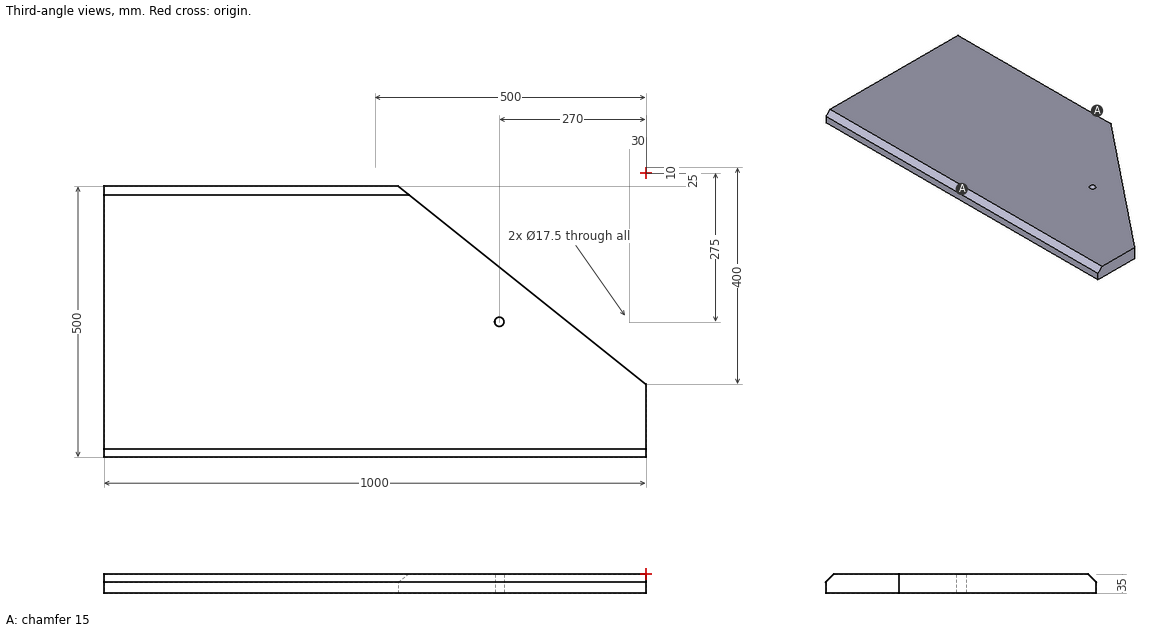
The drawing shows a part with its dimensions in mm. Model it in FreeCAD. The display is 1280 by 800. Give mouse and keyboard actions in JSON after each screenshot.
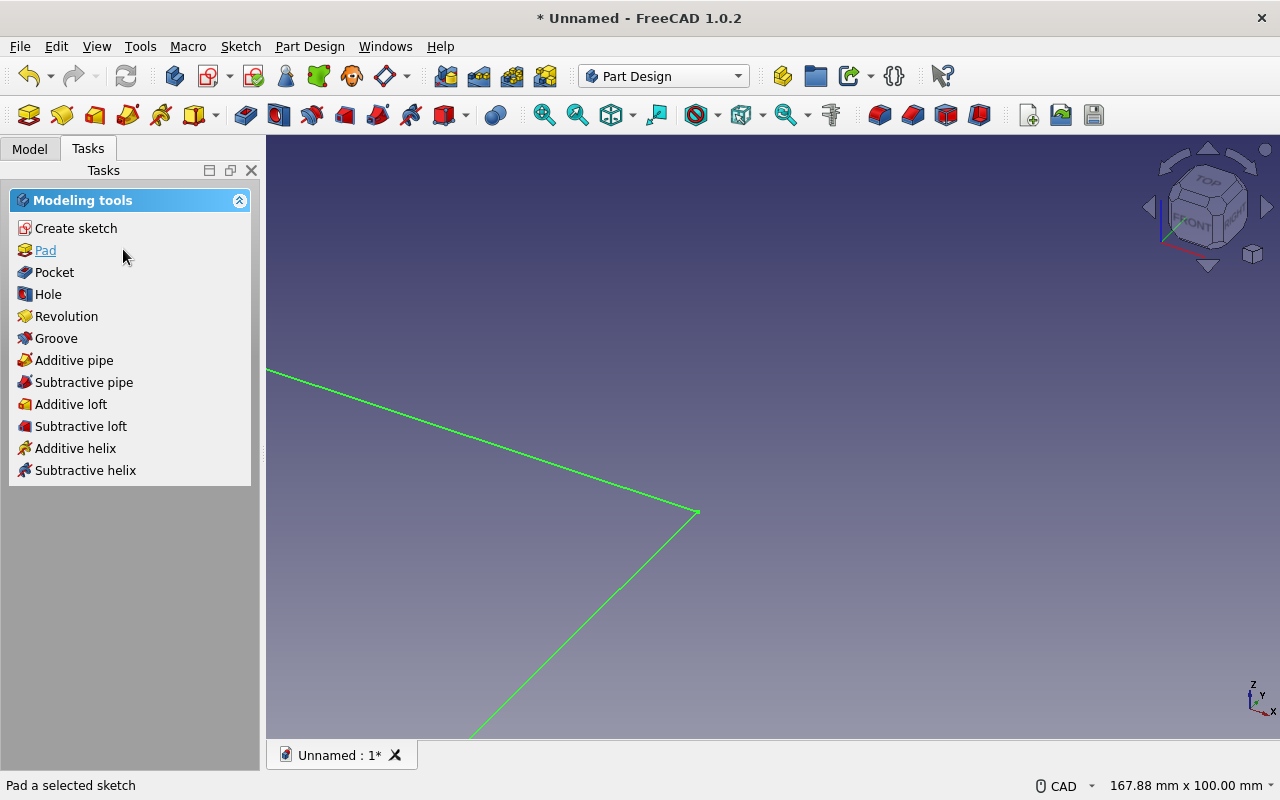
{"action": "left_click", "coordinate": [29, 116]}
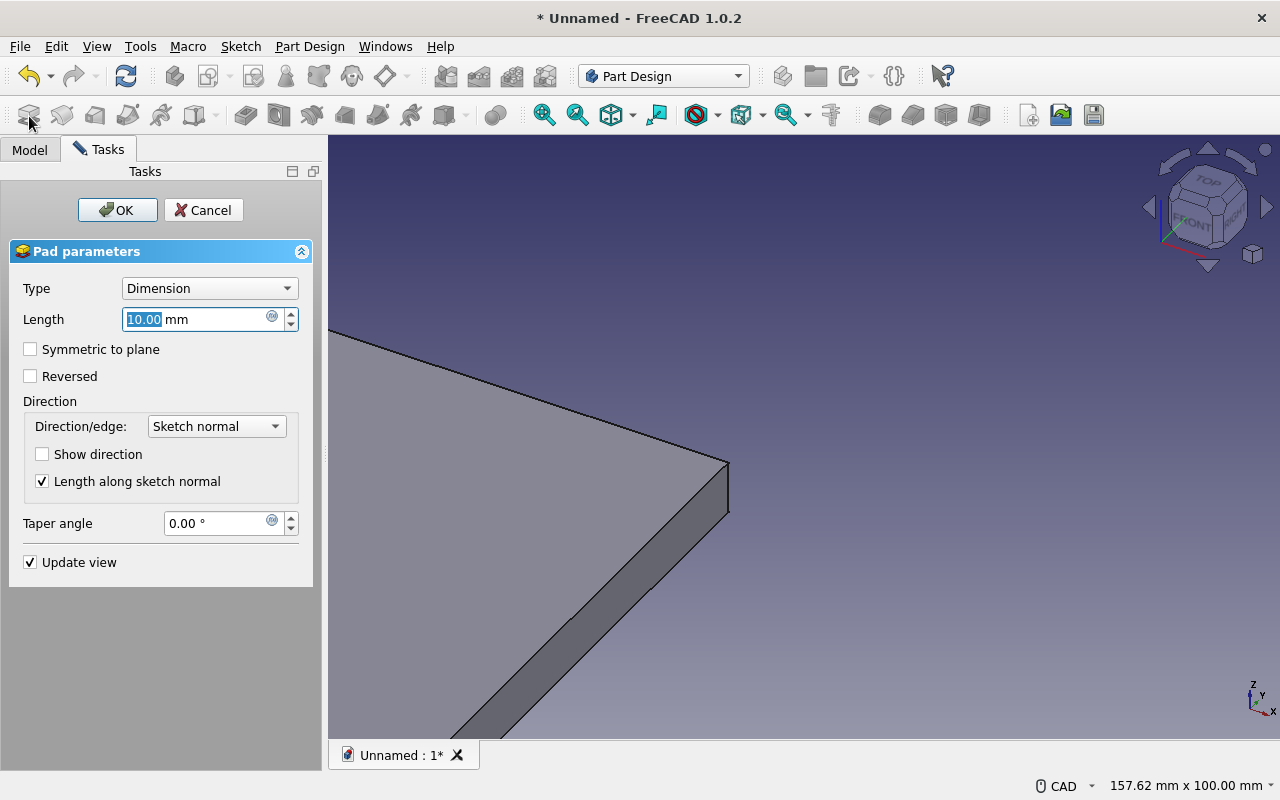
{"action": "type", "text": "35"}
{"action": "key", "text": "Tab"}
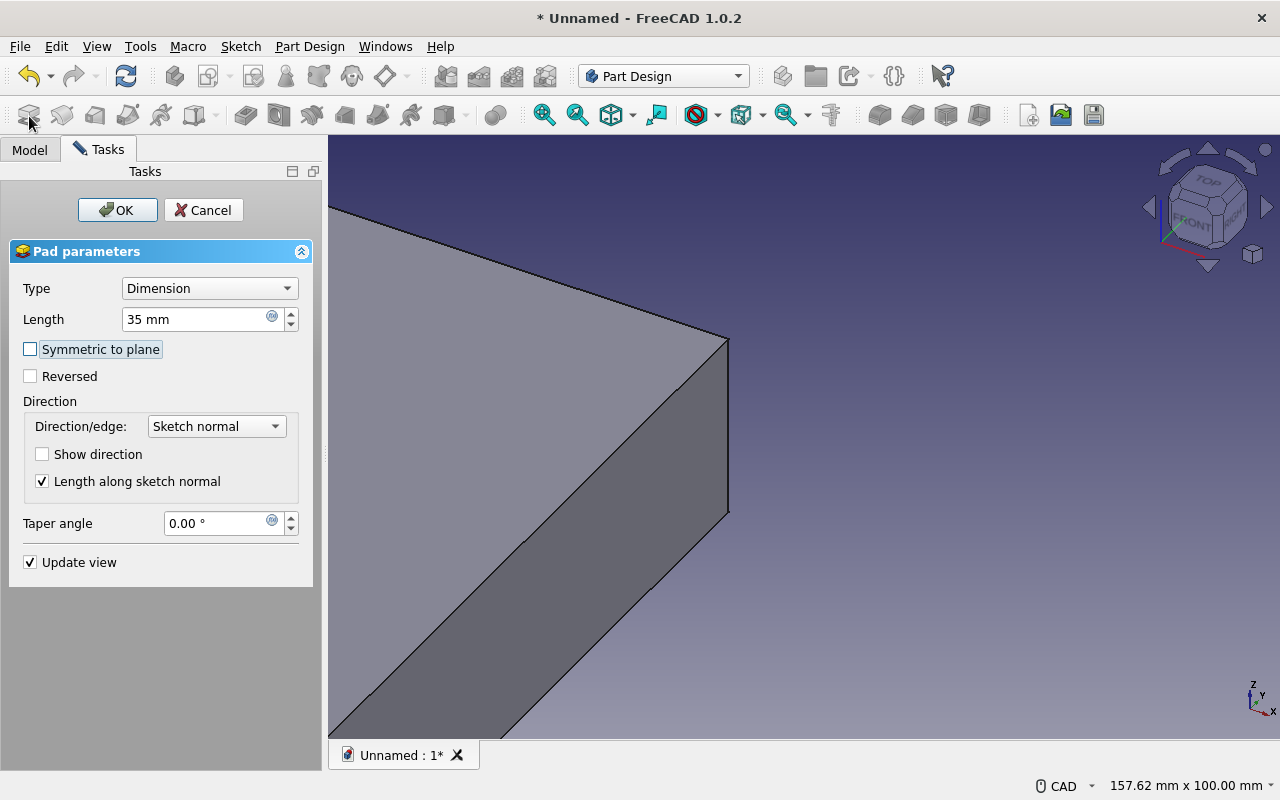
{"action": "left_click", "coordinate": [31, 376]}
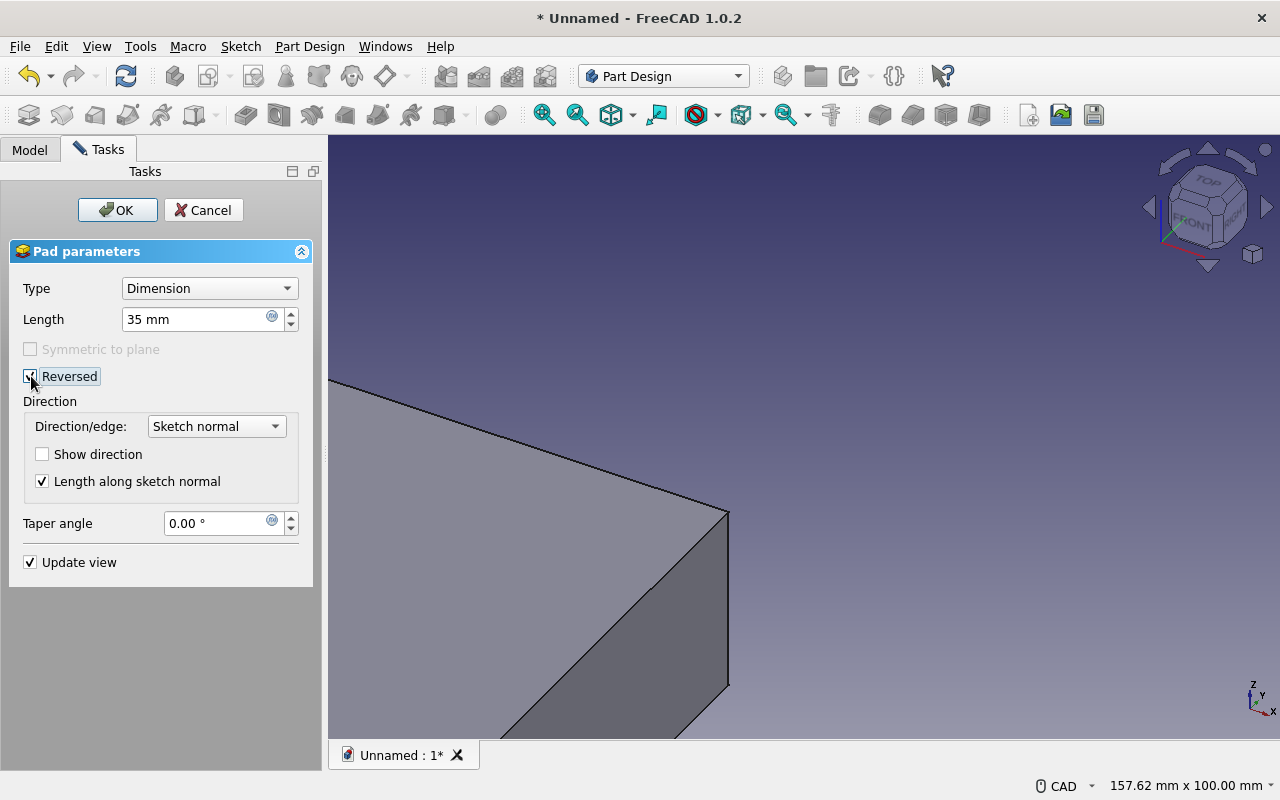
{"action": "left_click", "coordinate": [118, 210]}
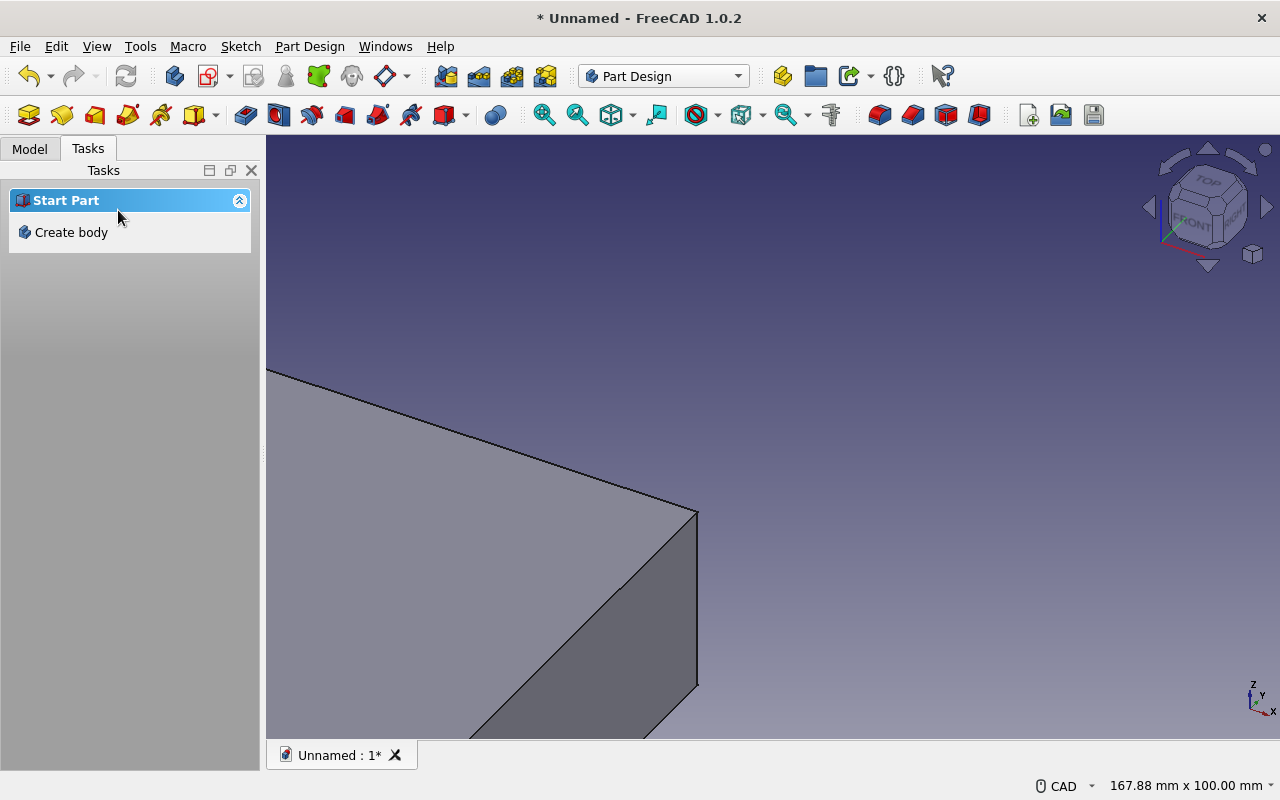
{"action": "key", "text": "v f"}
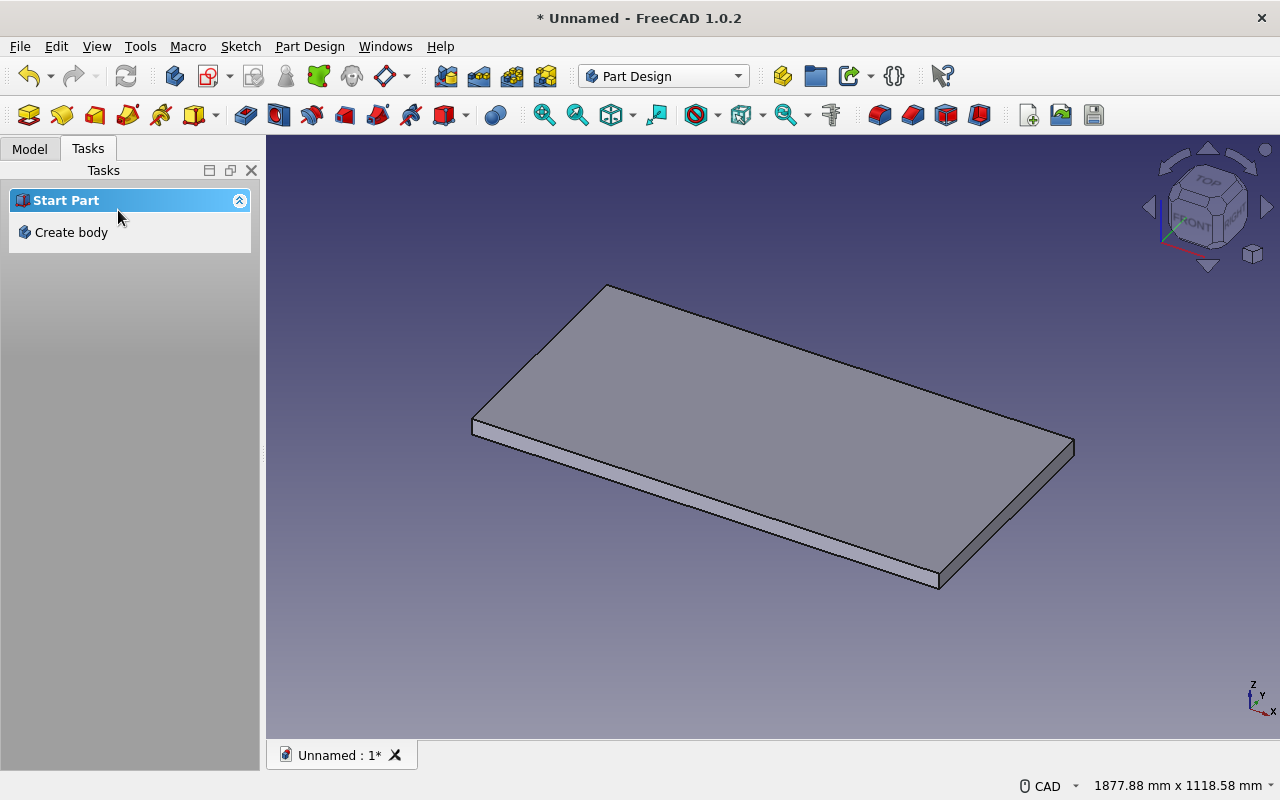
{"action": "left_click", "coordinate": [208, 76]}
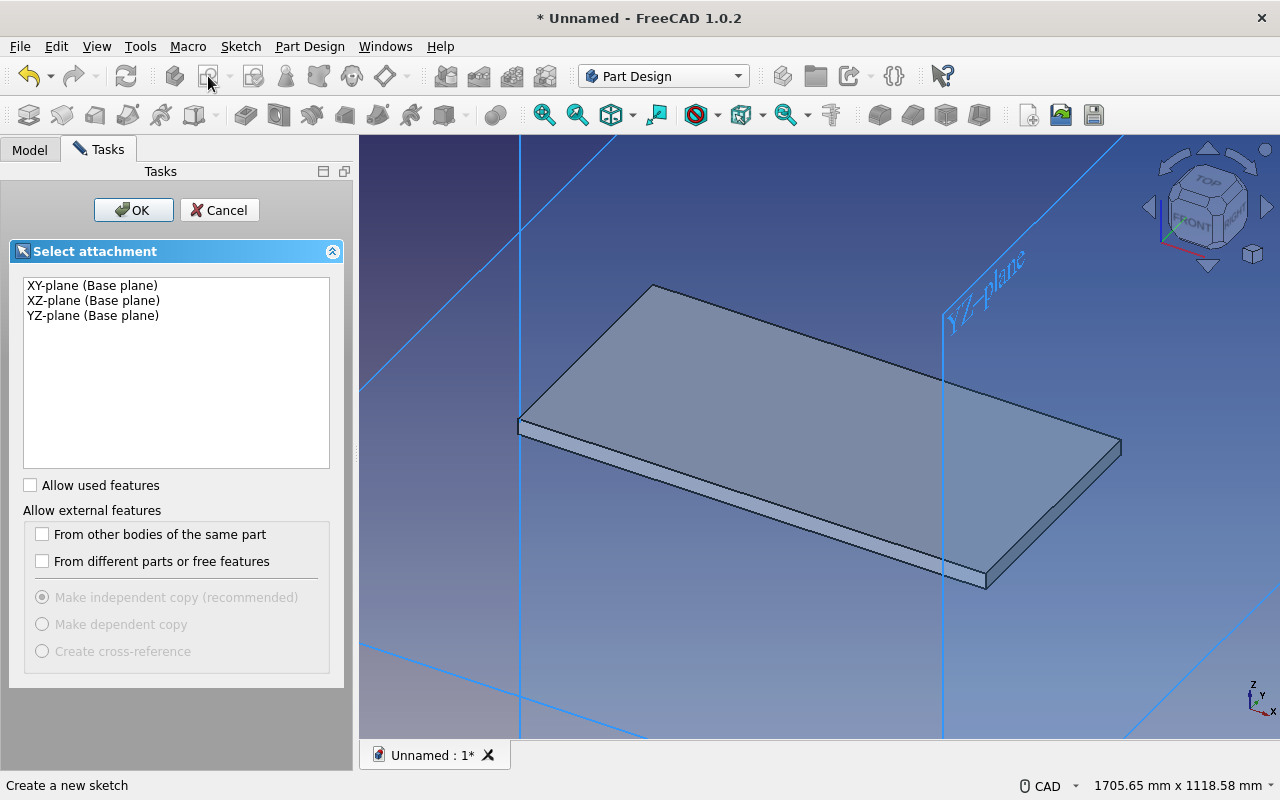
{"action": "left_click", "coordinate": [84, 286]}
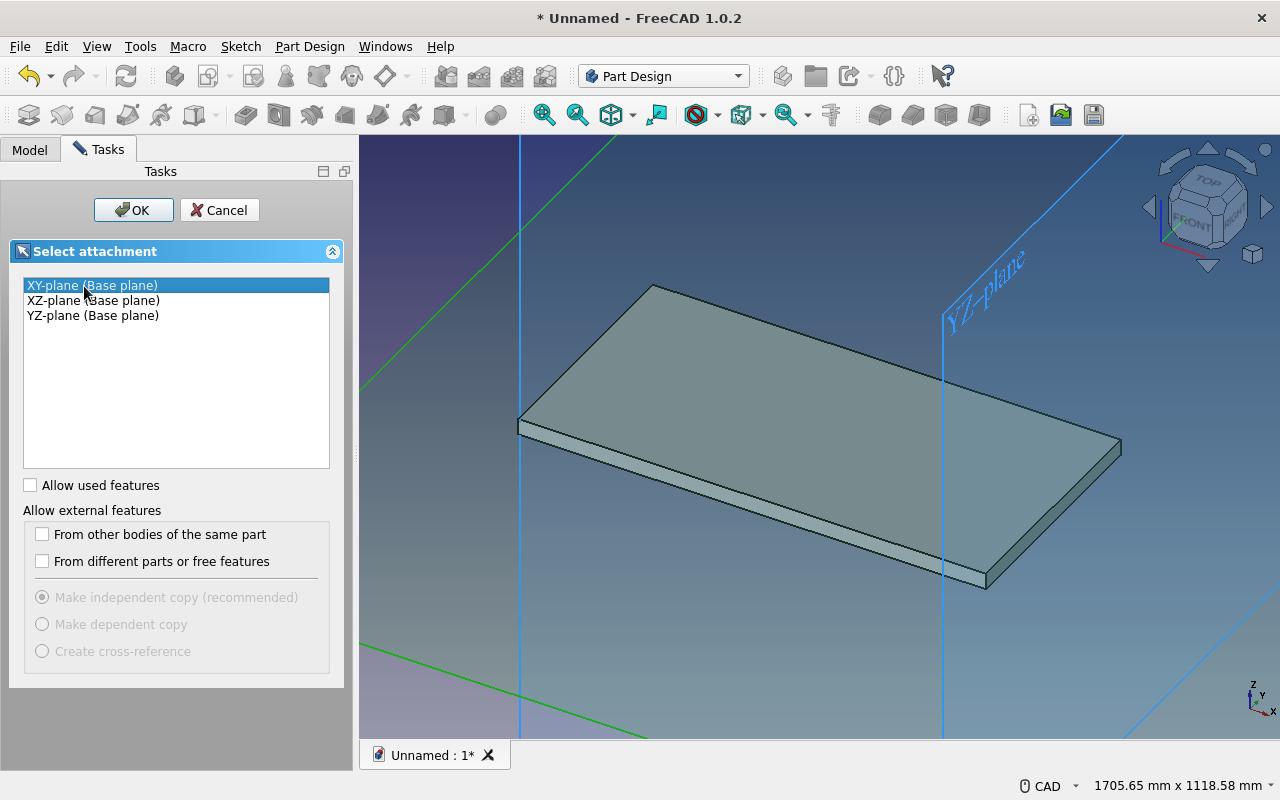
{"action": "left_click", "coordinate": [134, 210]}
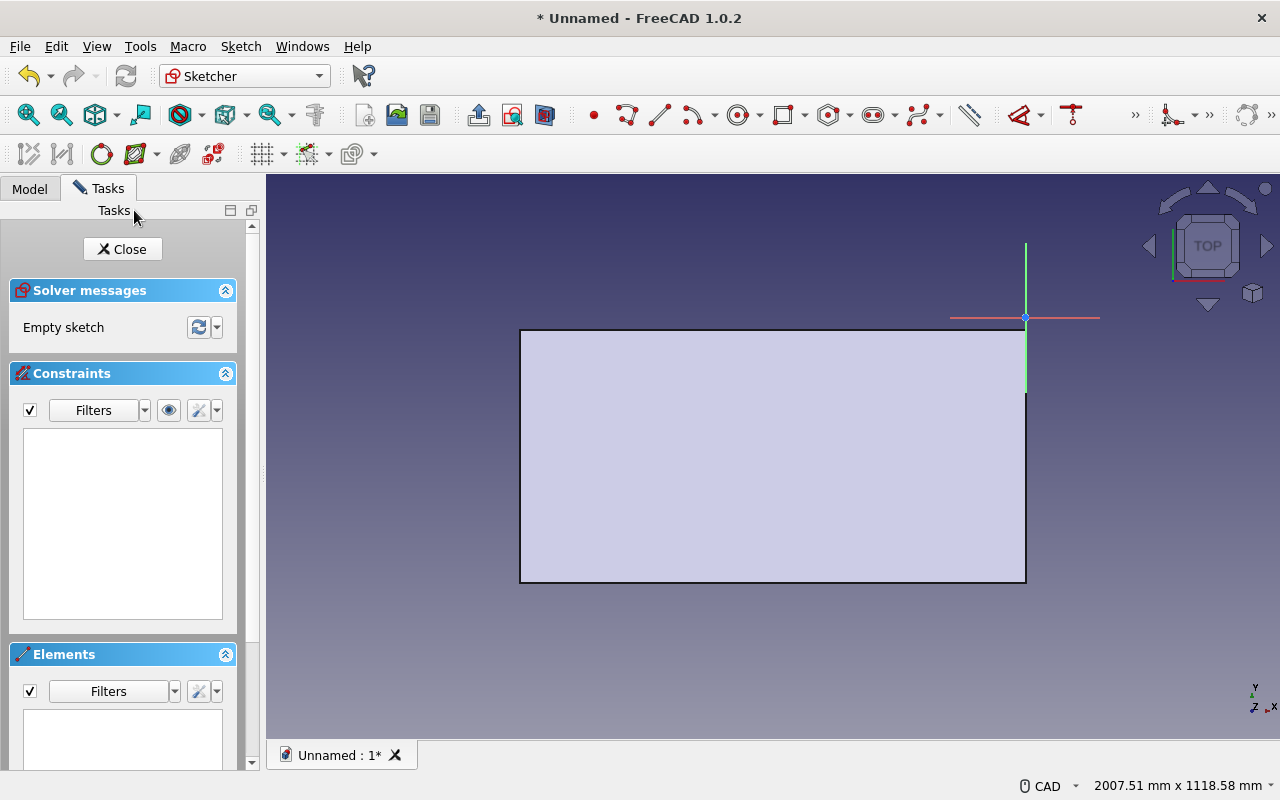
{"action": "scroll", "coordinate": [1101, 350], "scroll_direction": "up", "scroll_amount": 5}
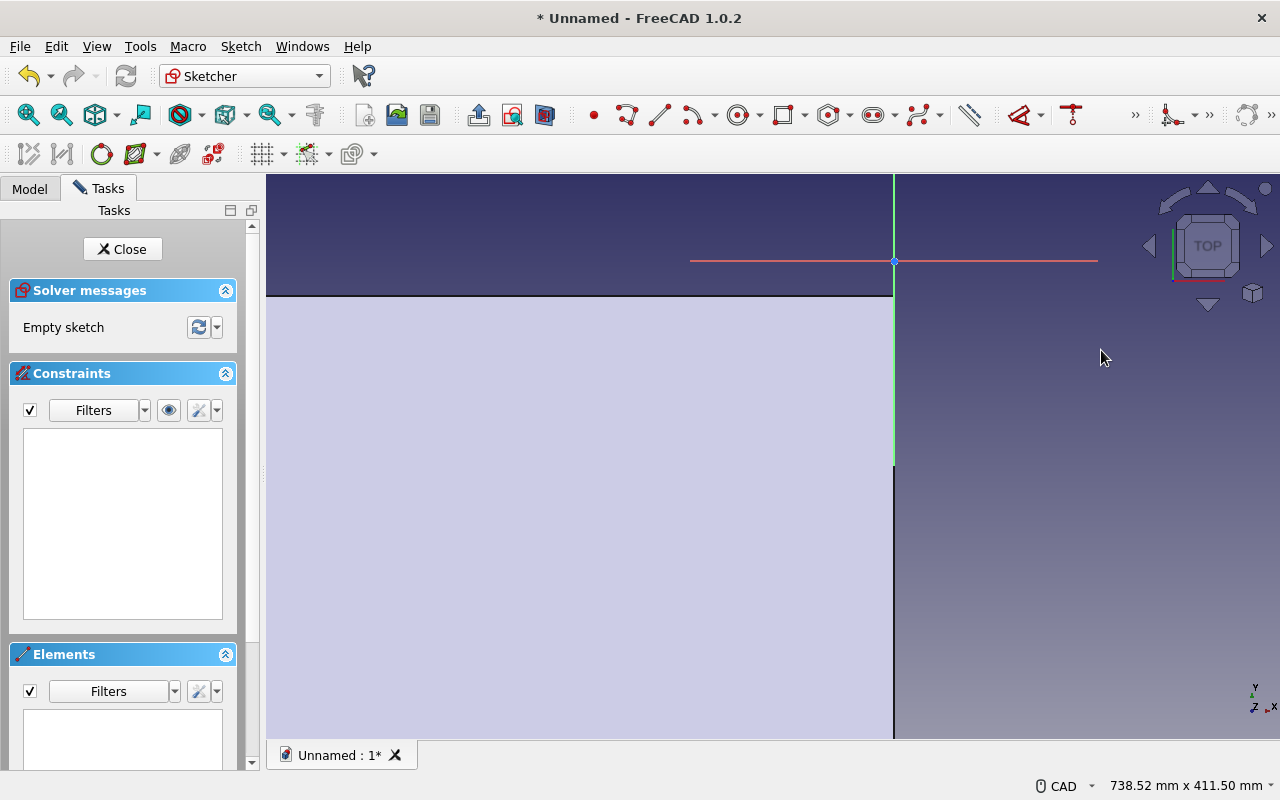
{"action": "key", "text": "g c"}